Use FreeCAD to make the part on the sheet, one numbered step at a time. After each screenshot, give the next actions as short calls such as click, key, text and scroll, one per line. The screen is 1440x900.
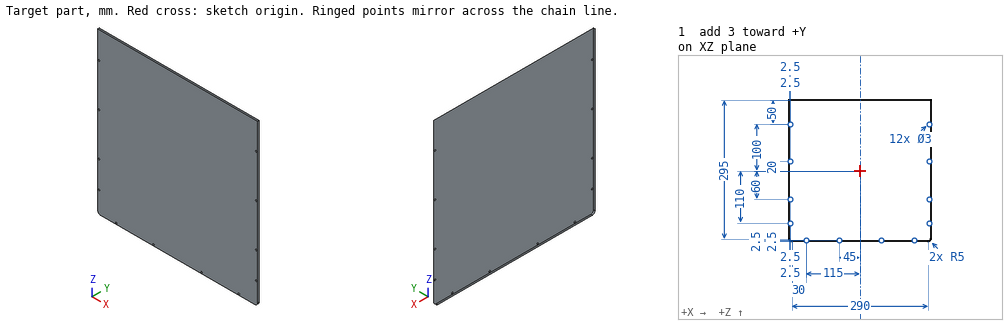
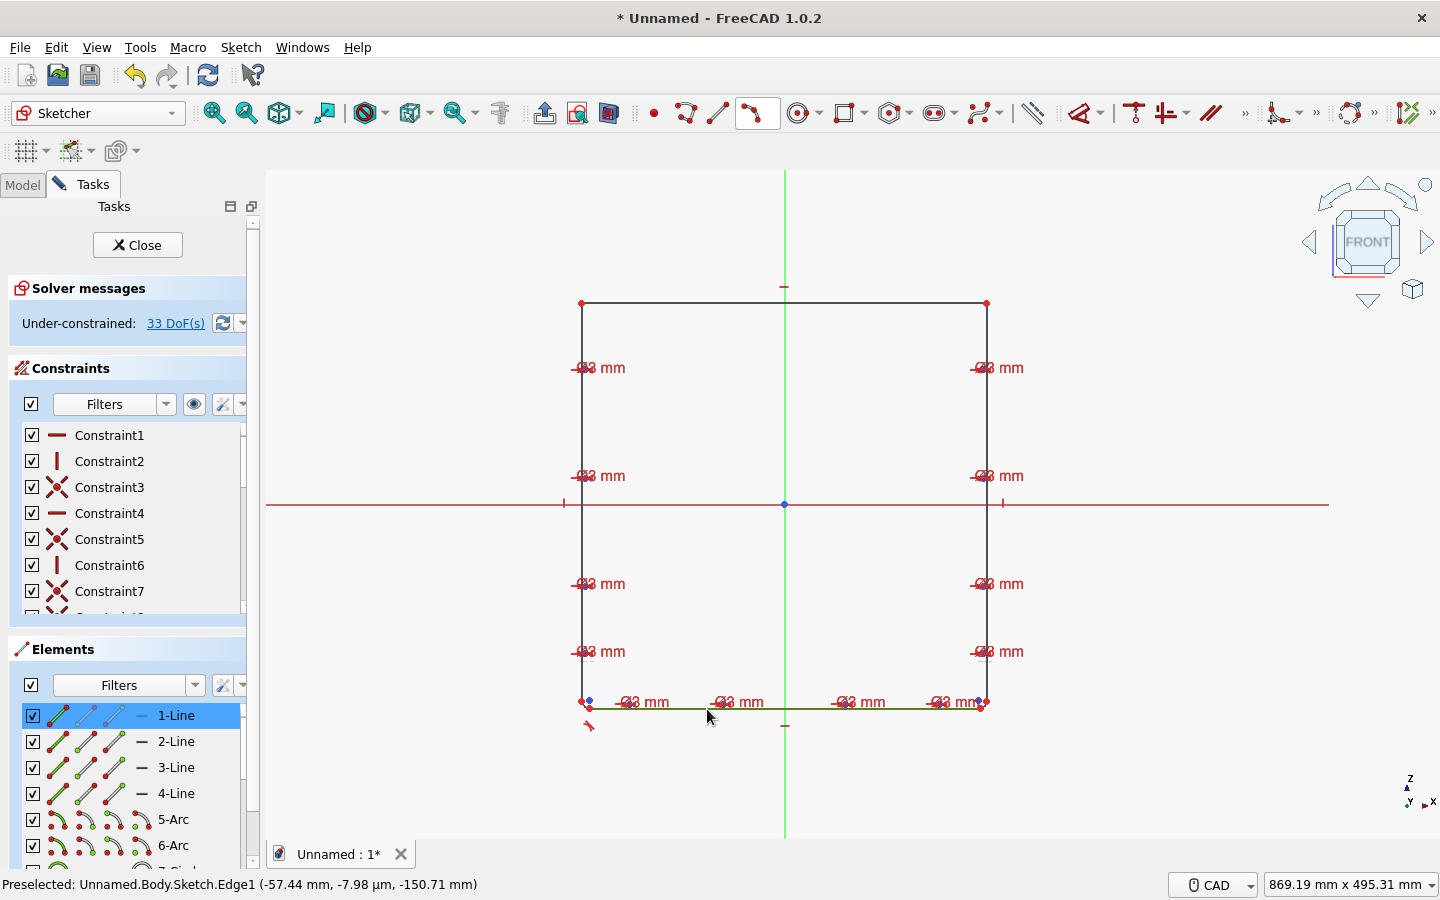
scroll(985, 706, up, 6)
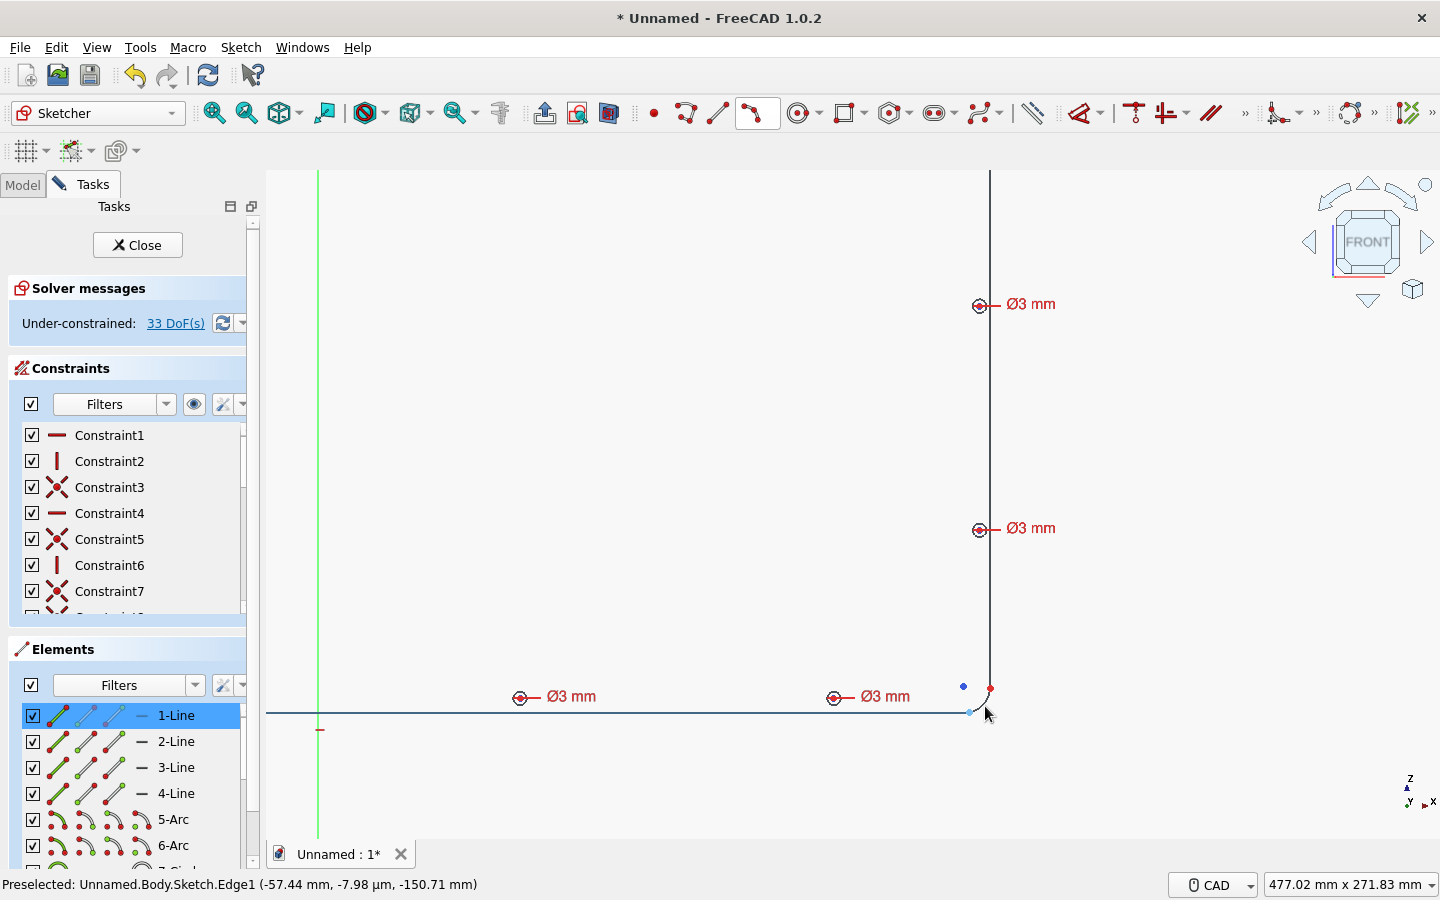
click(984, 704)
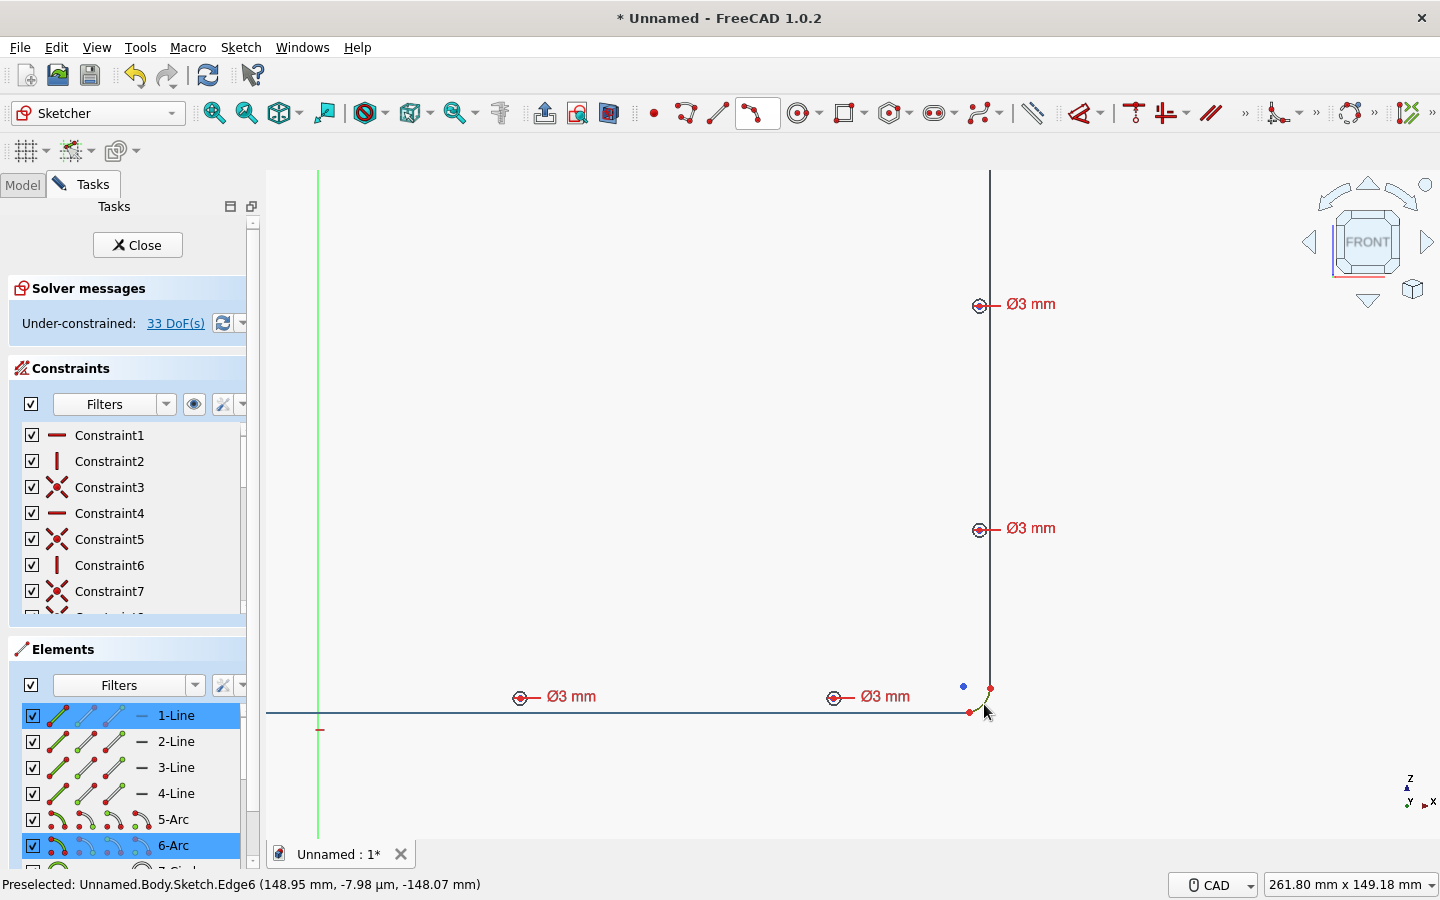
key(t)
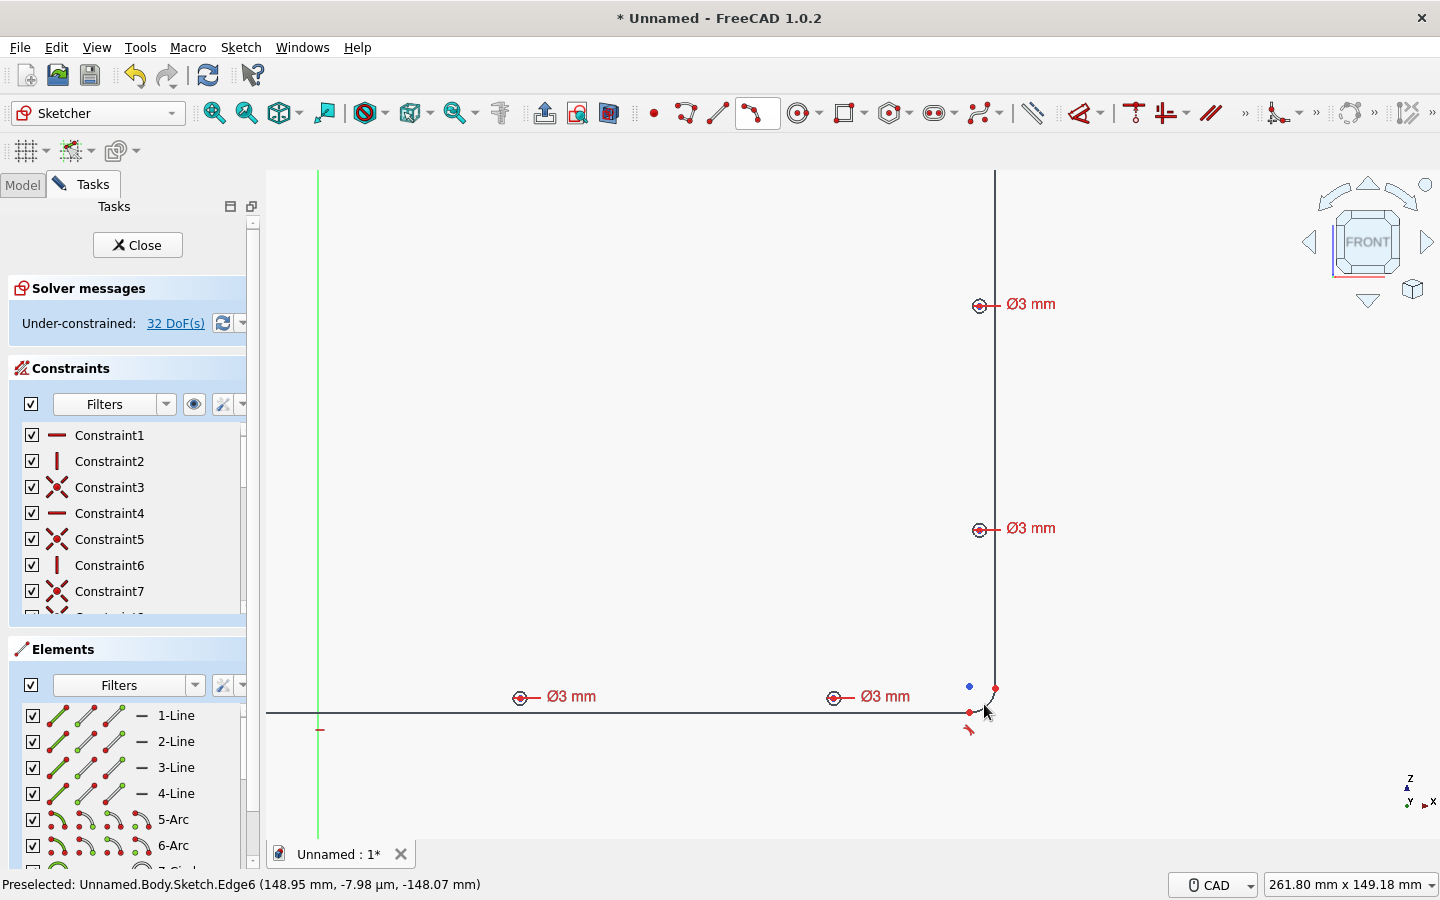
scroll(985, 706, down, 6)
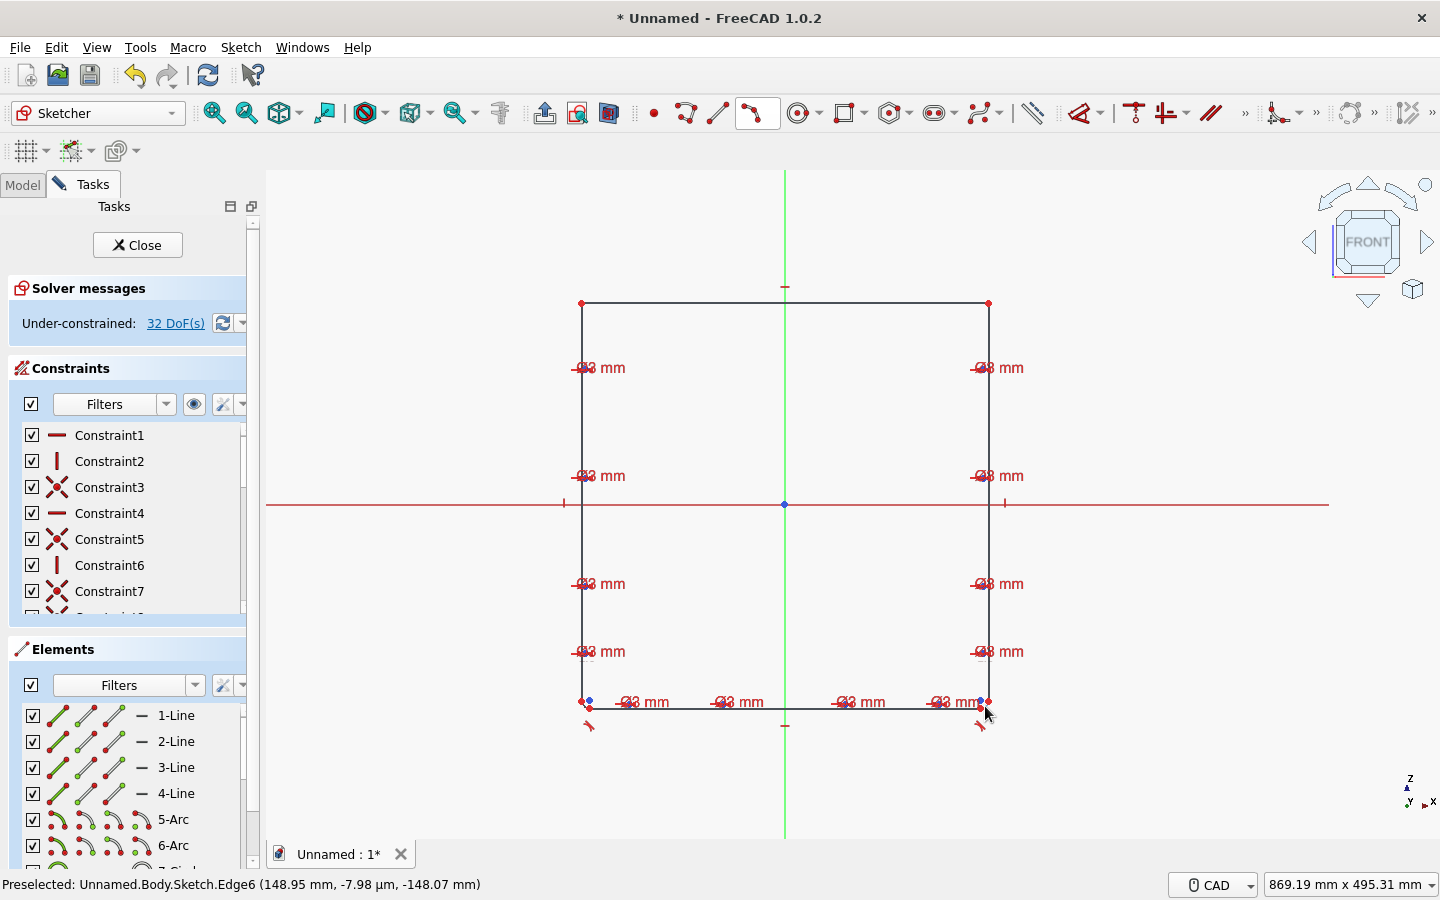
scroll(582, 582, up, 7)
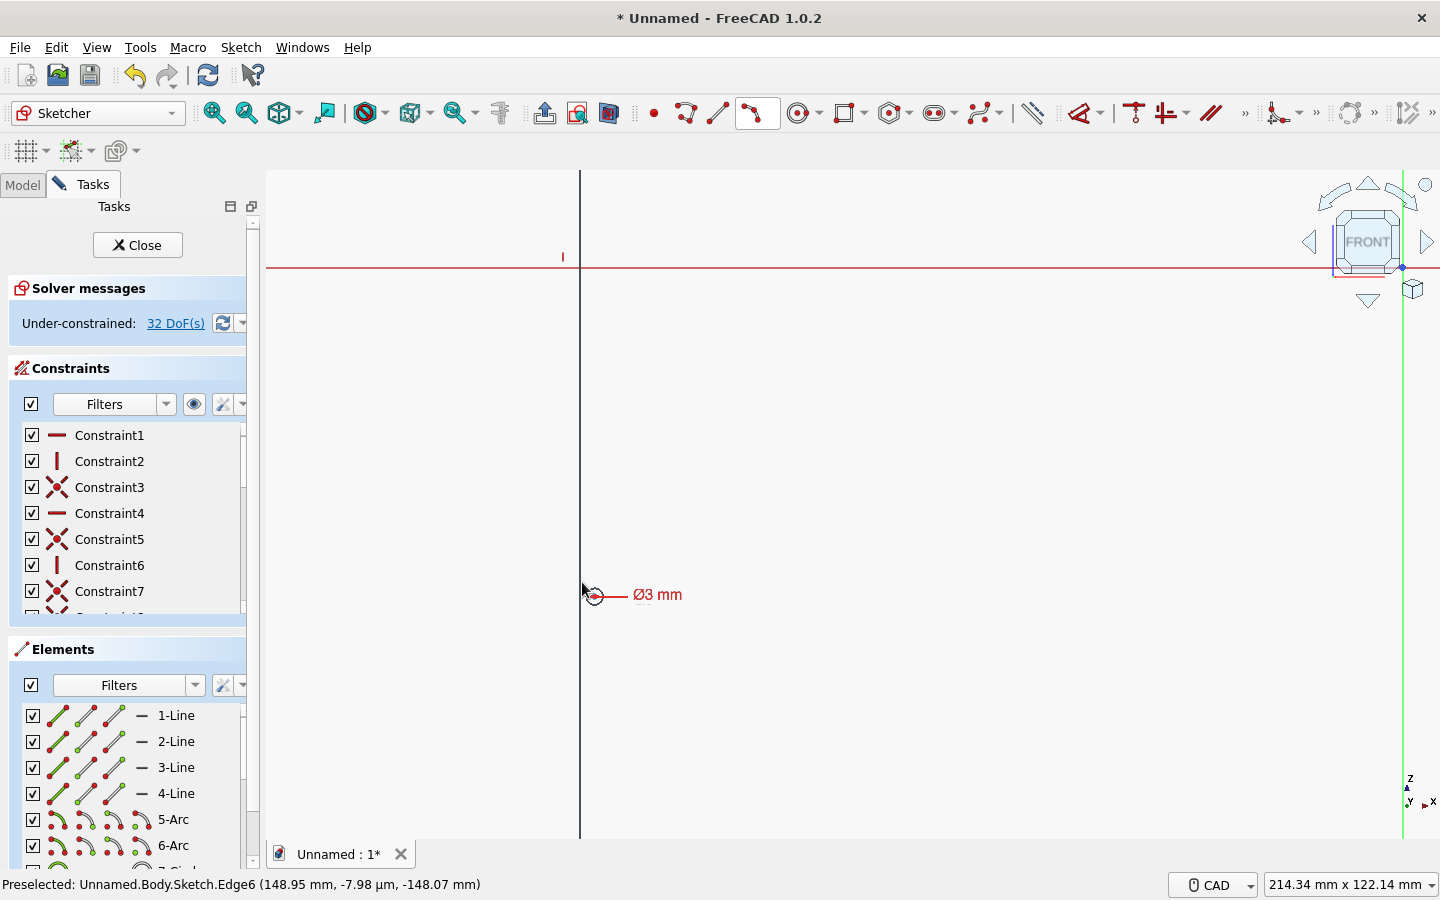
click(580, 580)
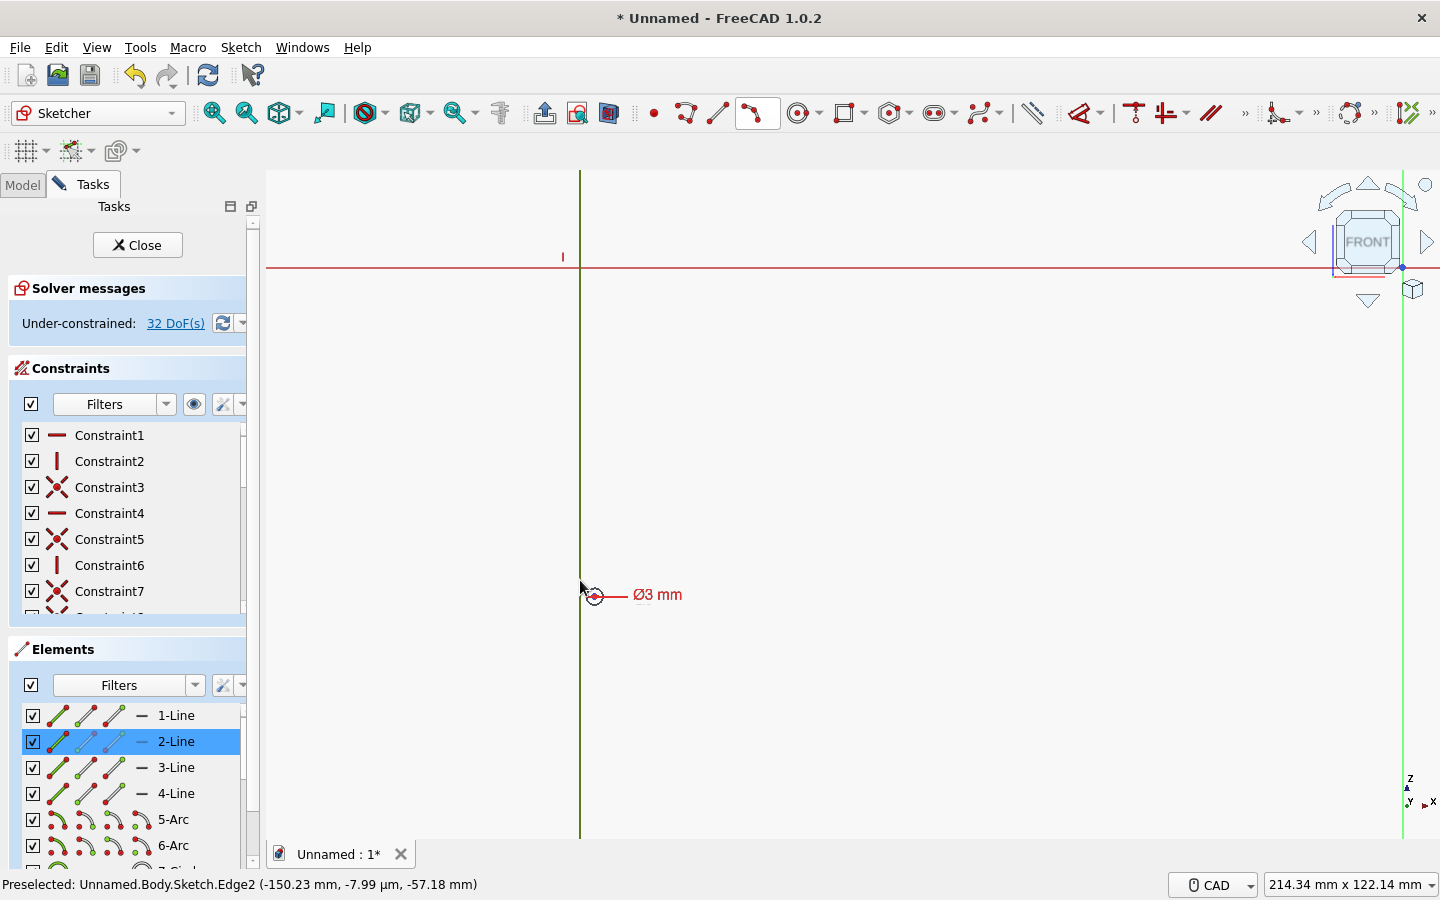
scroll(582, 582, down, 7)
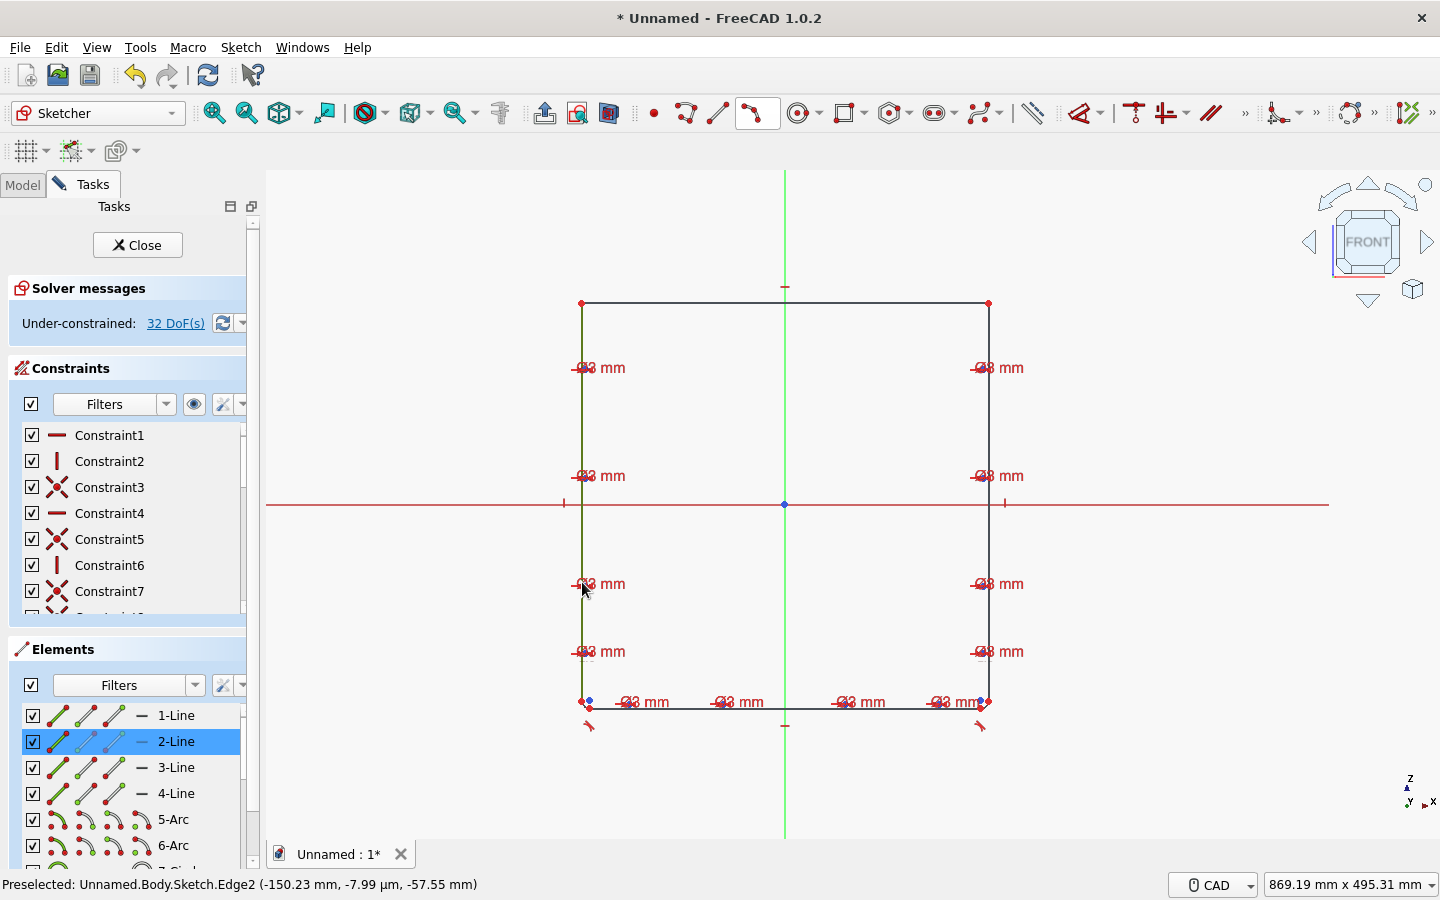
scroll(583, 705, up, 7)